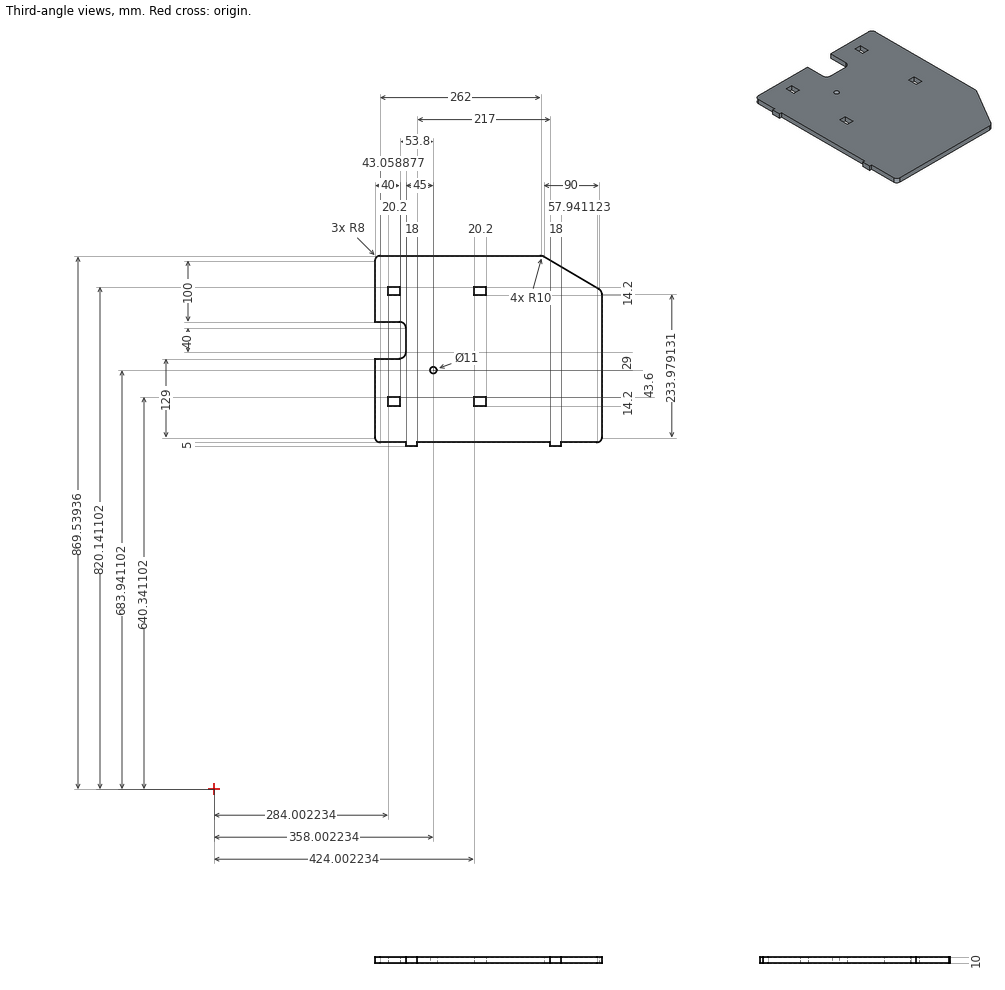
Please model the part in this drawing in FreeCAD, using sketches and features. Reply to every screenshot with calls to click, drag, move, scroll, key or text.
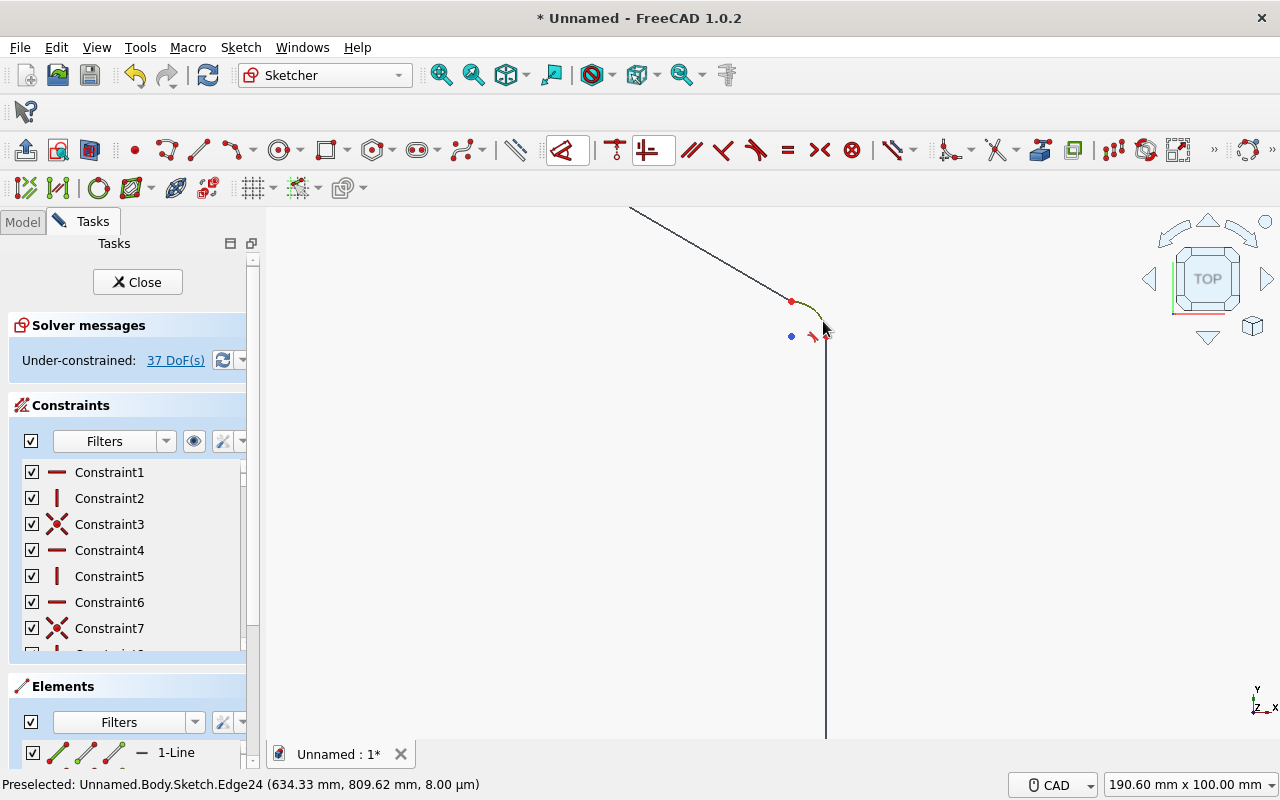
click(788, 150)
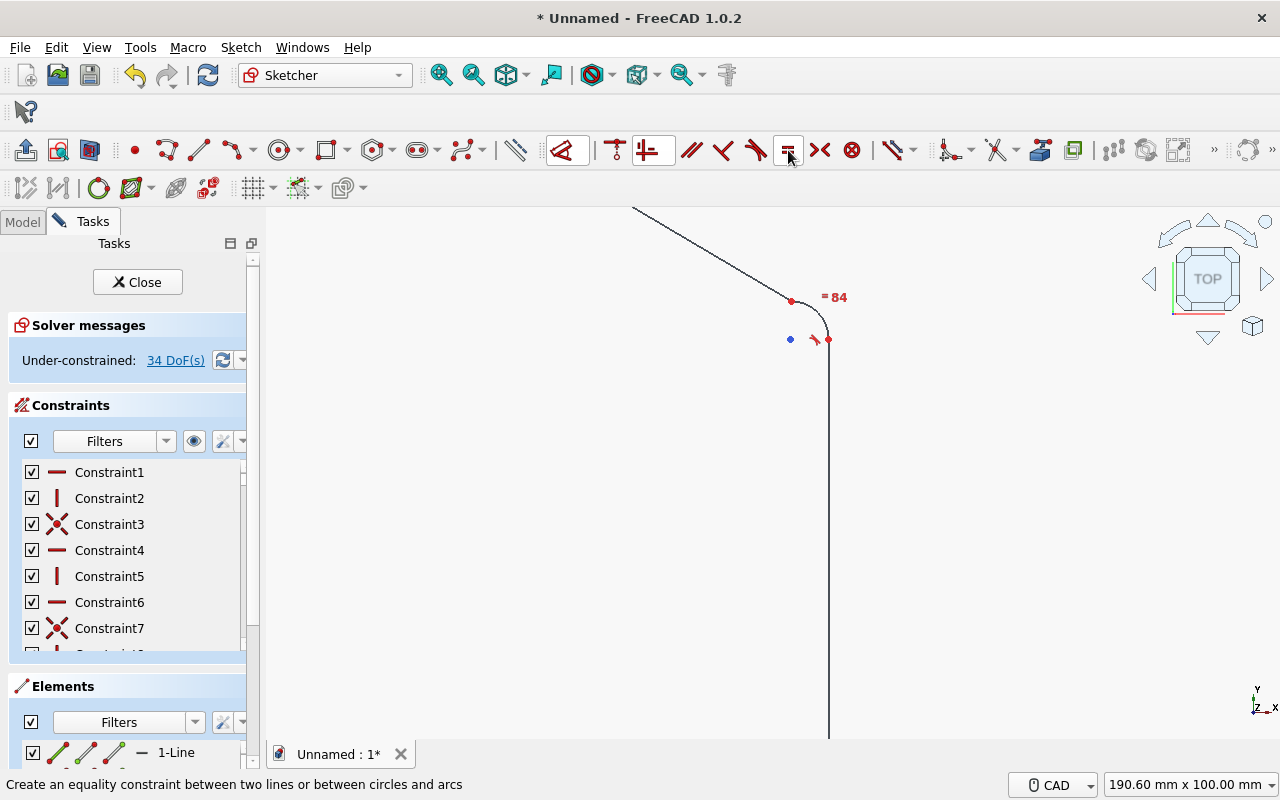
scroll(831, 325, down, 13)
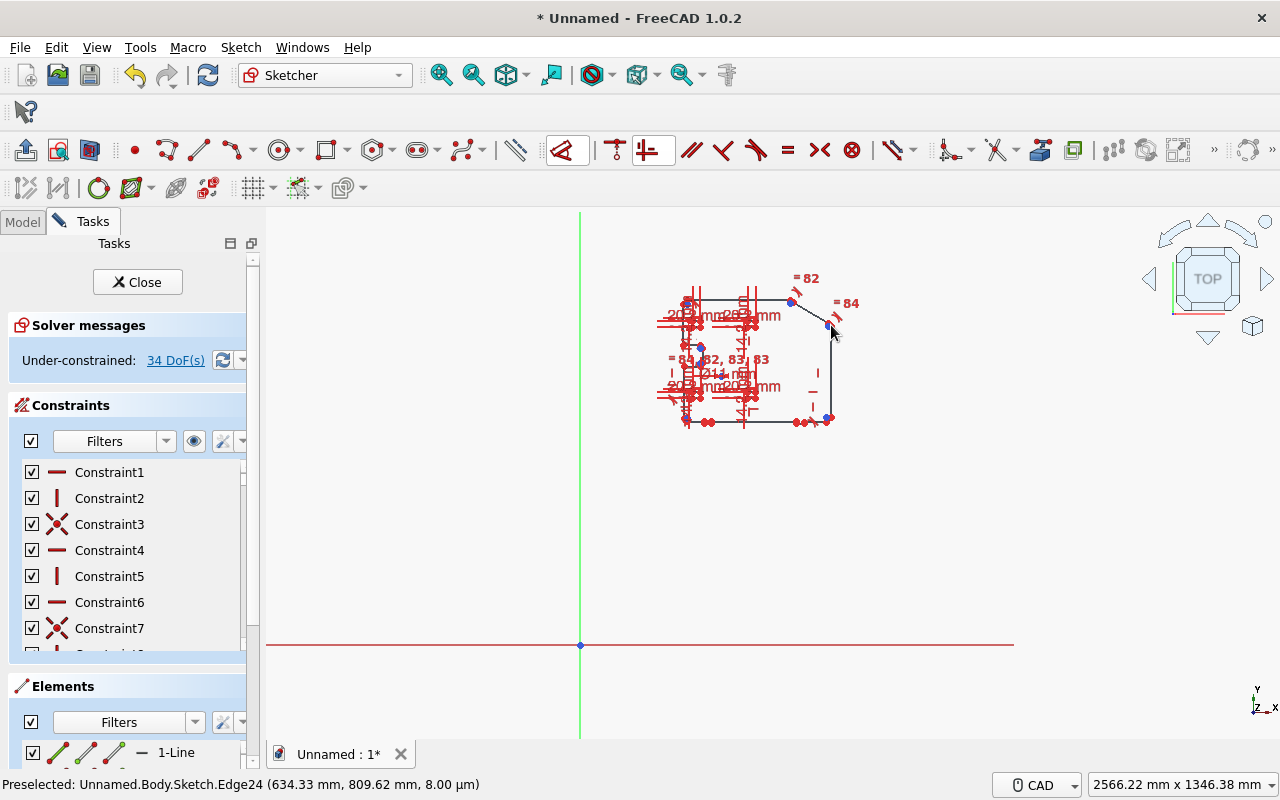
scroll(686, 301, up, 11)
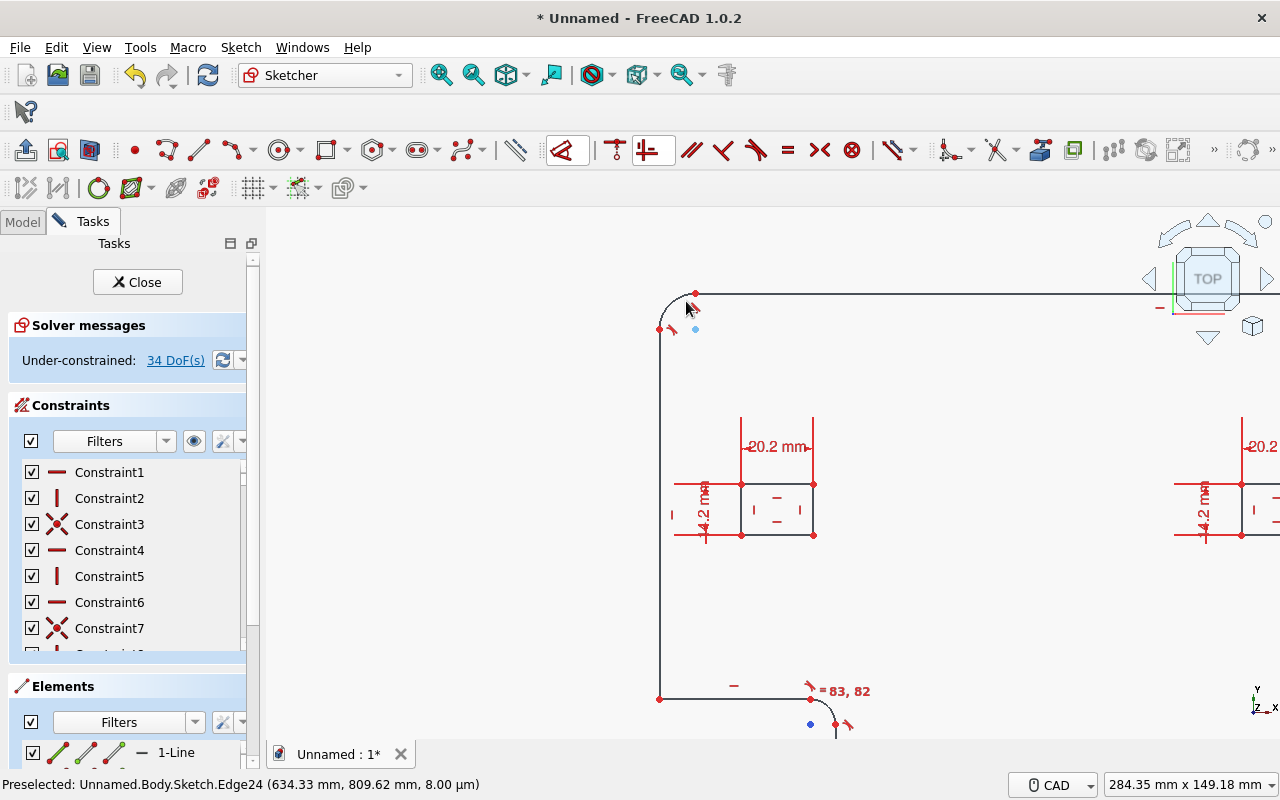
click(679, 298)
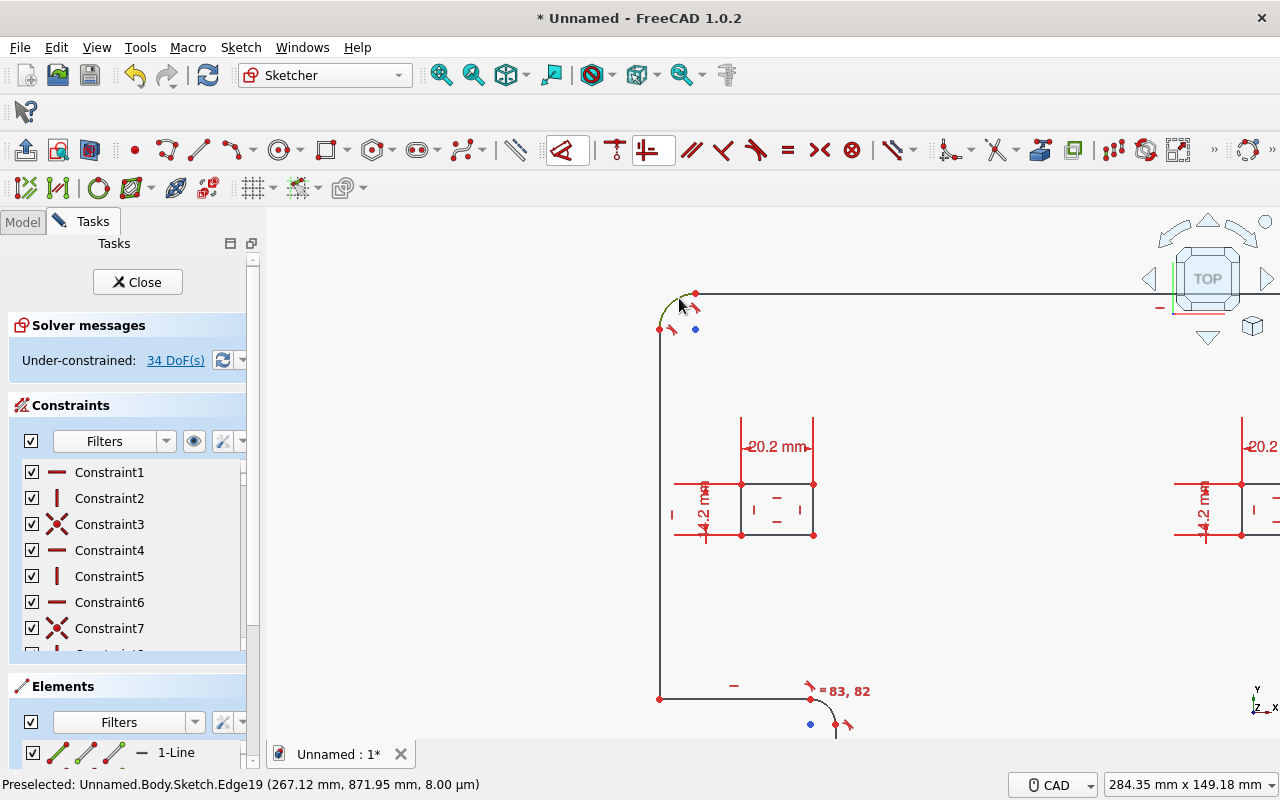
scroll(685, 301, down, 11)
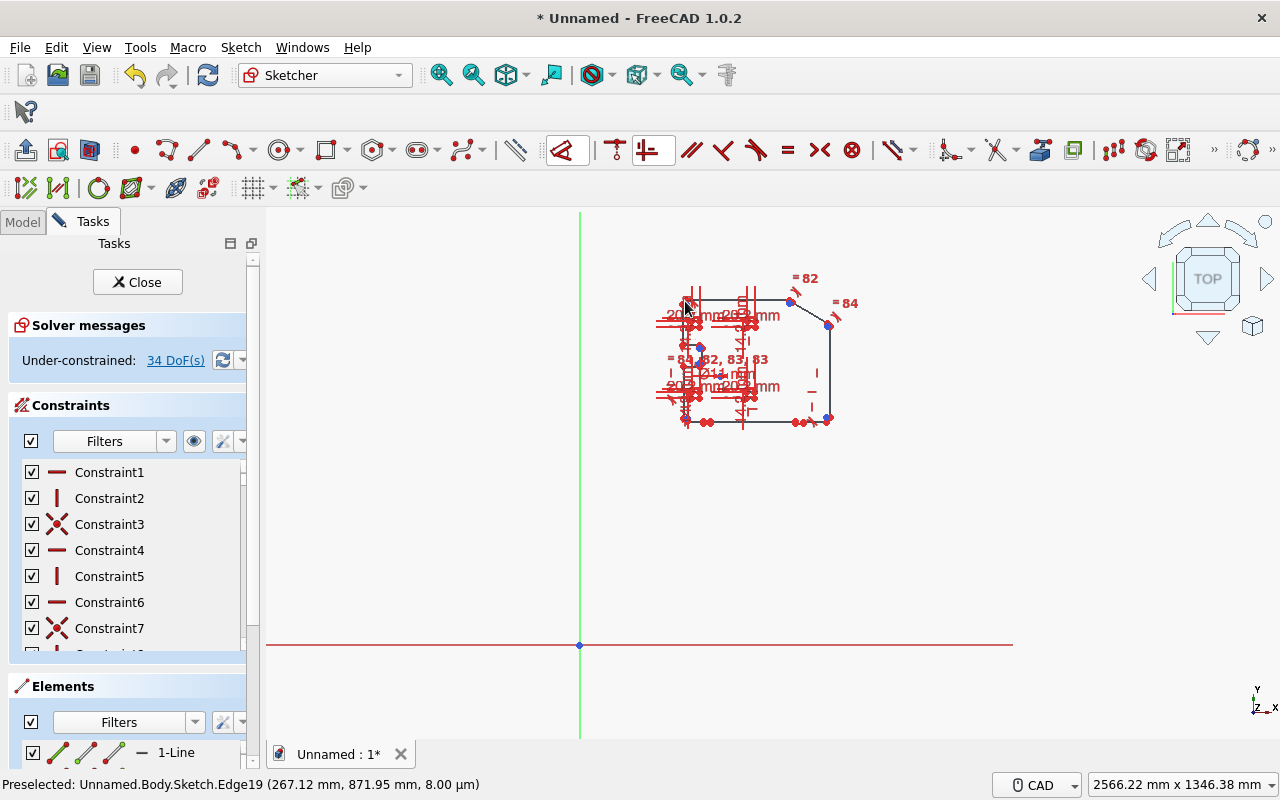
scroll(684, 420, up, 11)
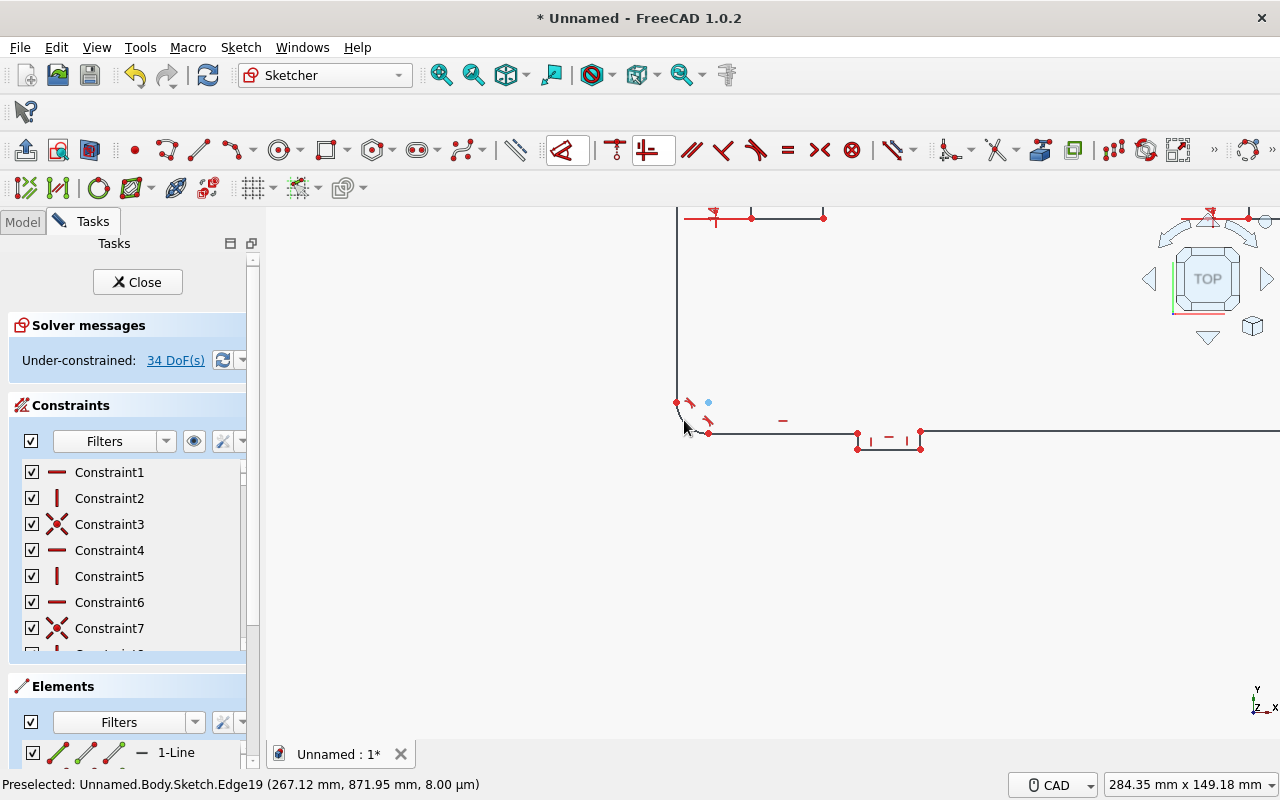
click(680, 417)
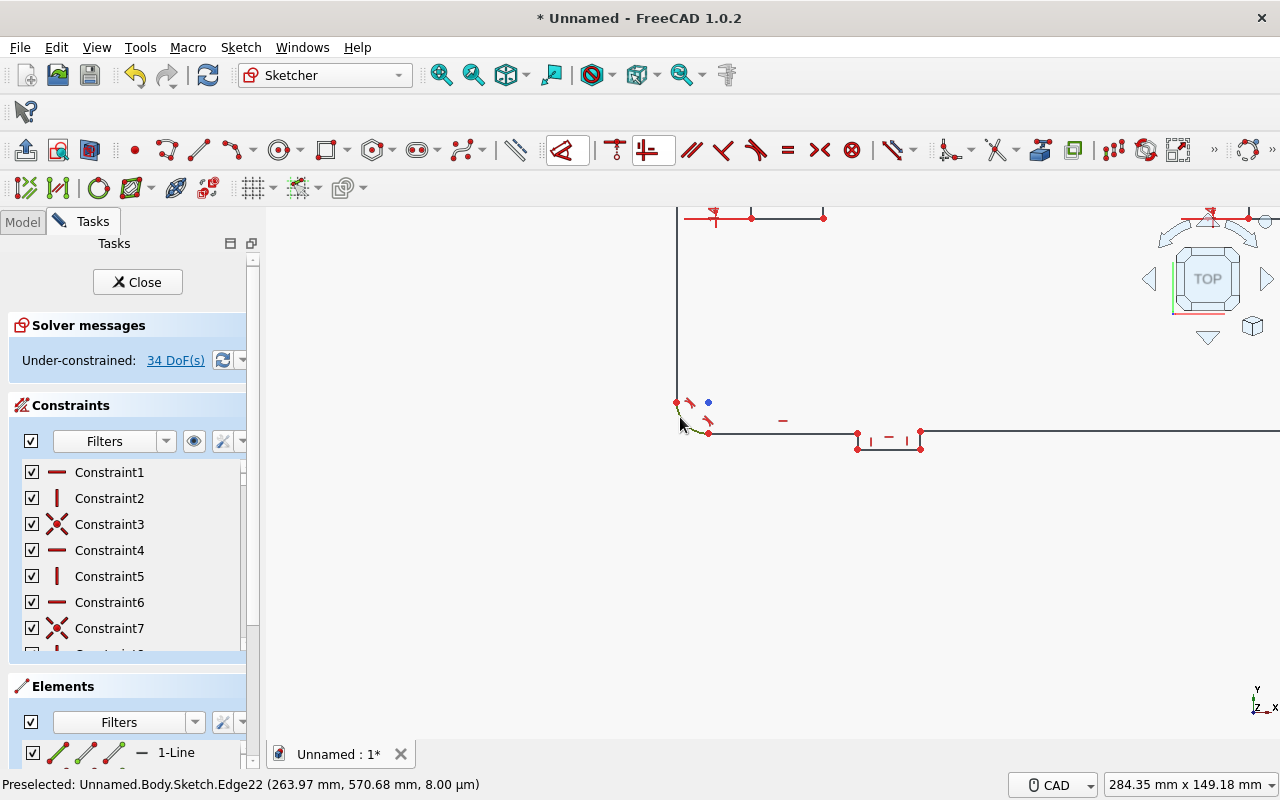
scroll(684, 420, down, 11)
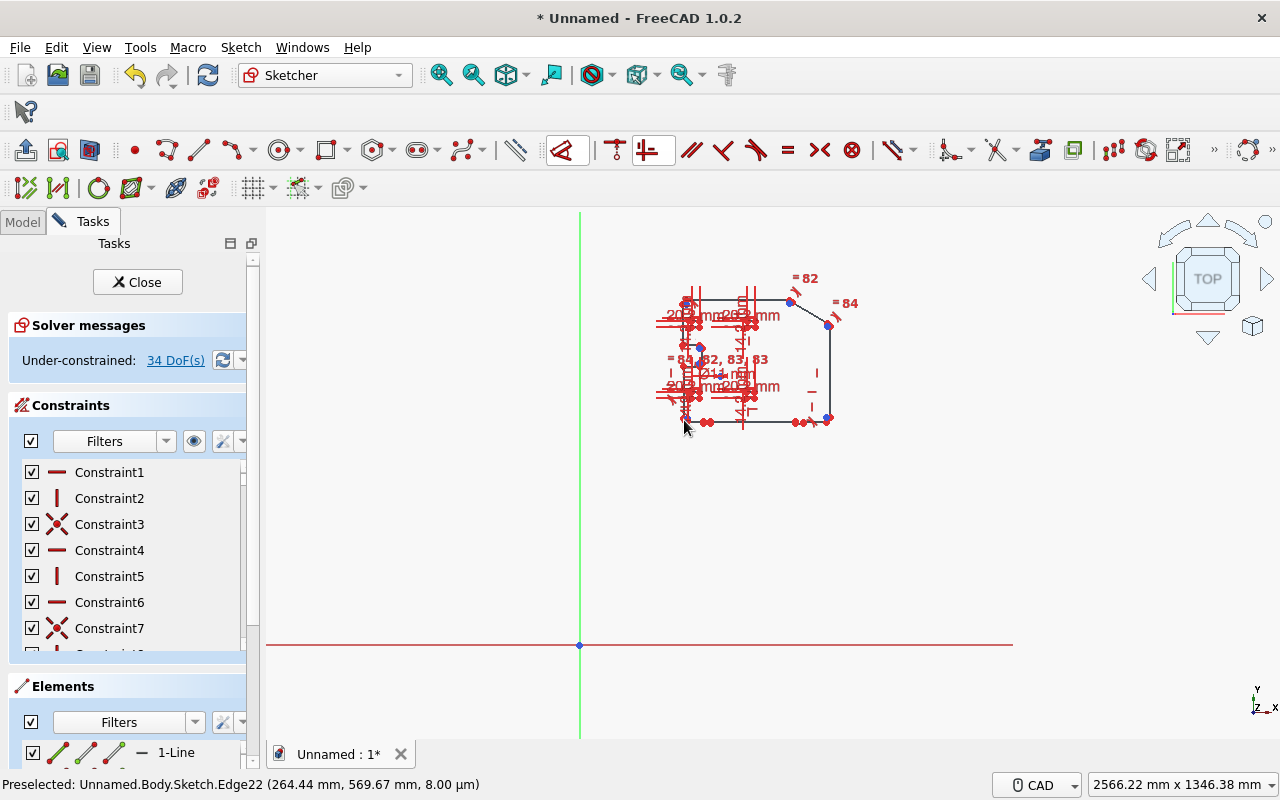
scroll(828, 422, up, 10)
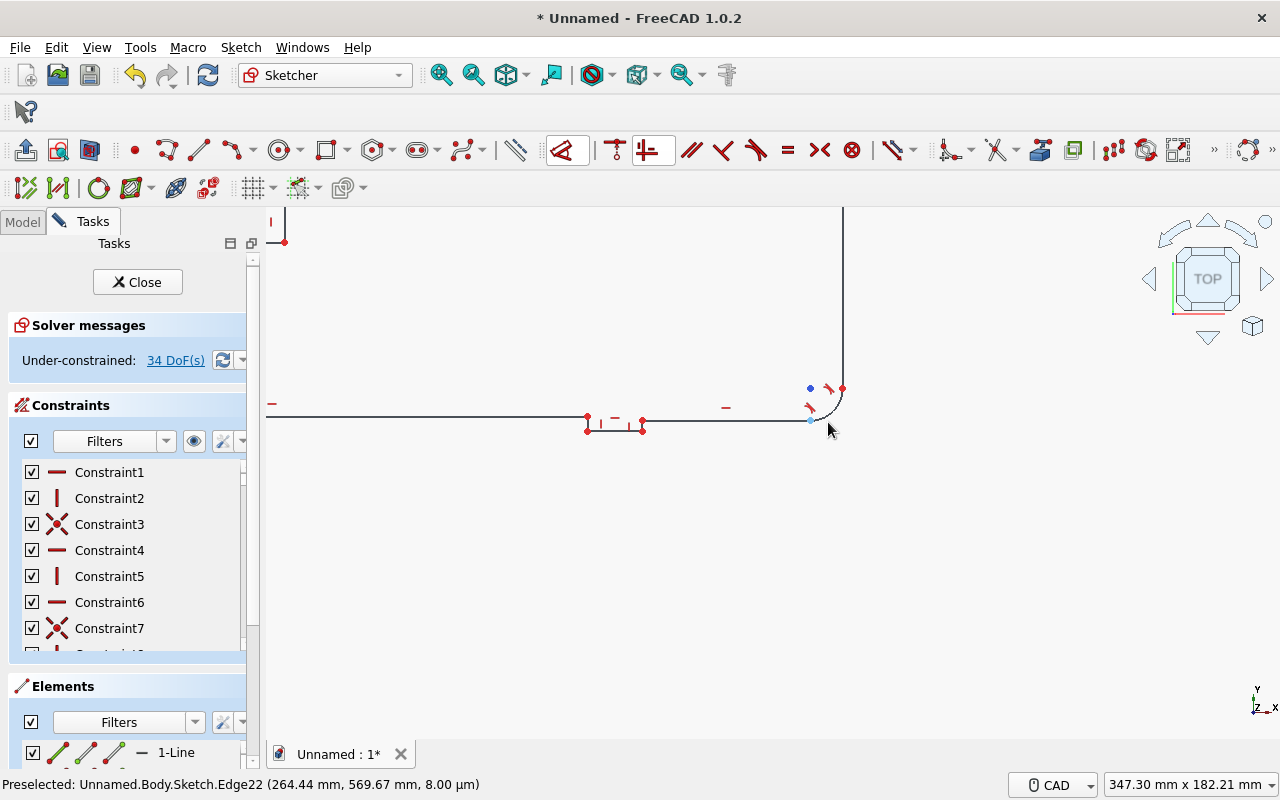
click(825, 417)